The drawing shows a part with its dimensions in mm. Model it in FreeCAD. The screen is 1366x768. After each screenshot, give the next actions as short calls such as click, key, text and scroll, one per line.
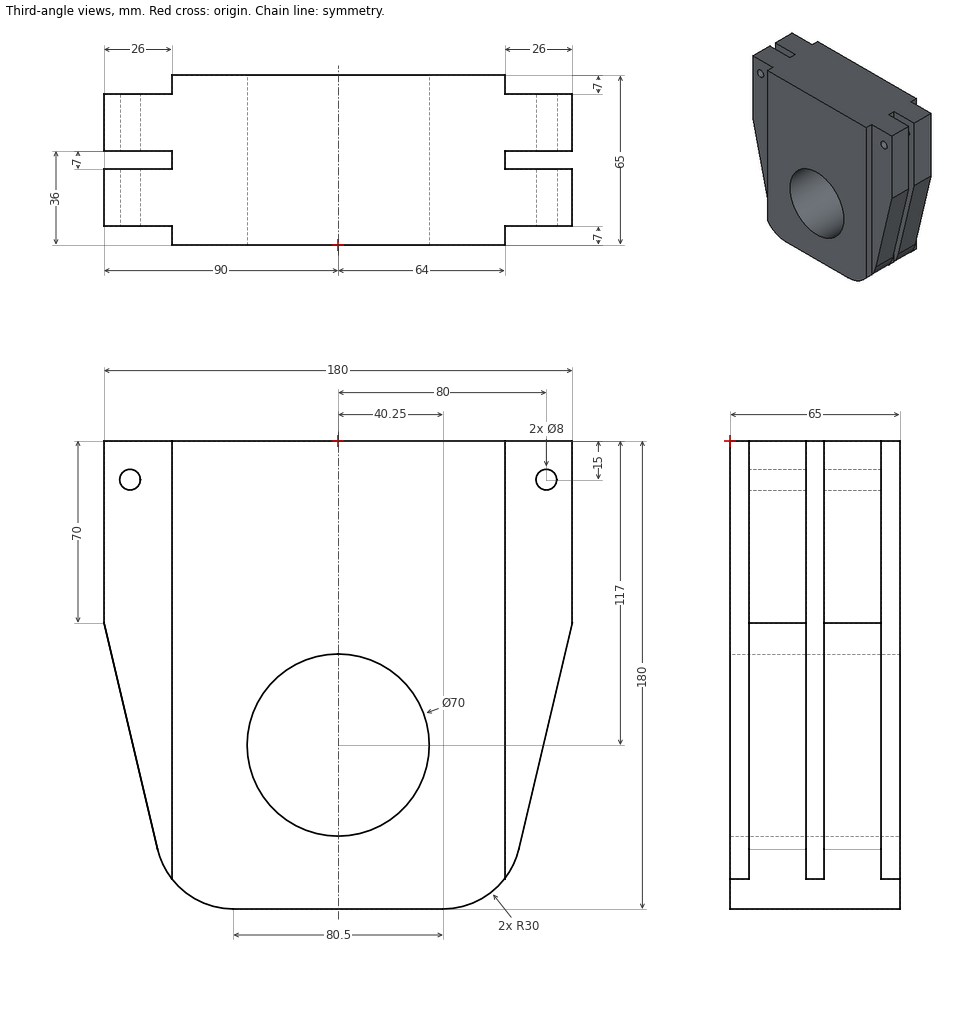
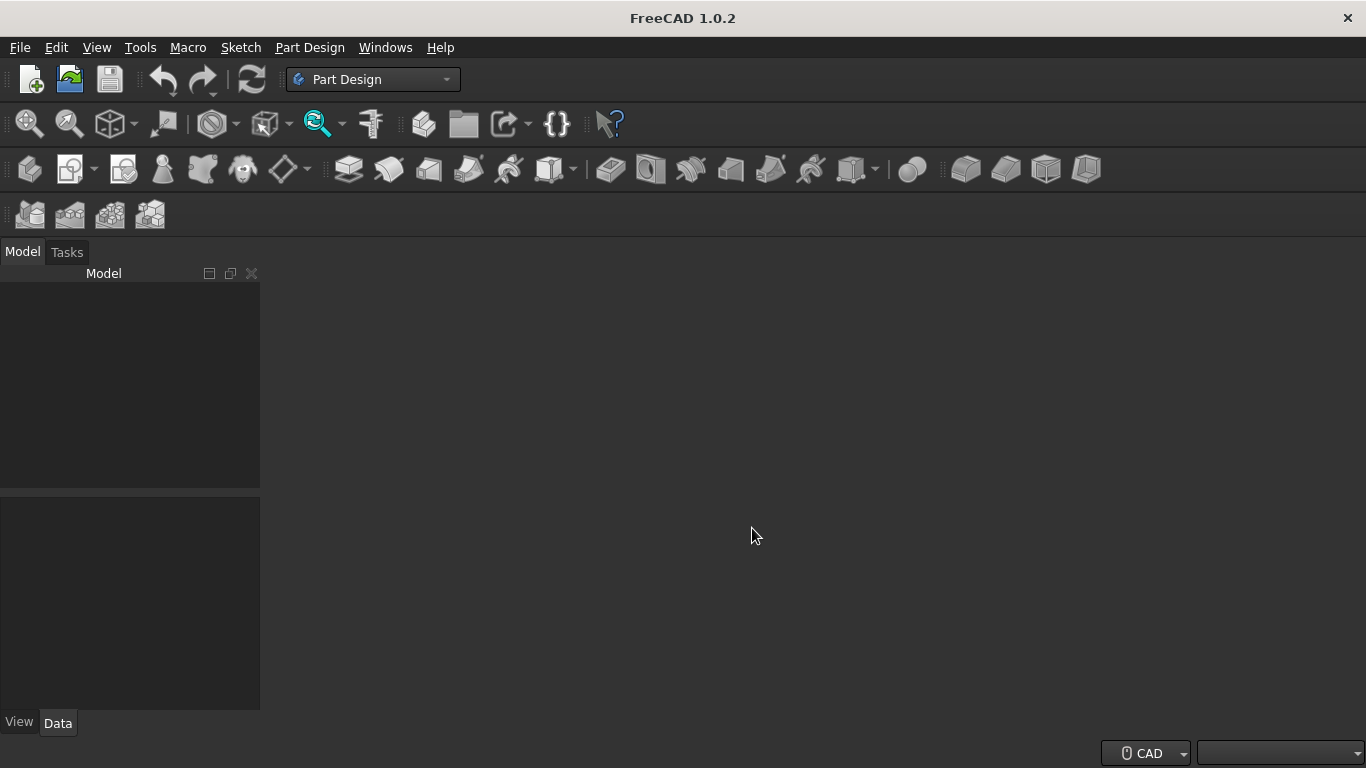
click(30, 80)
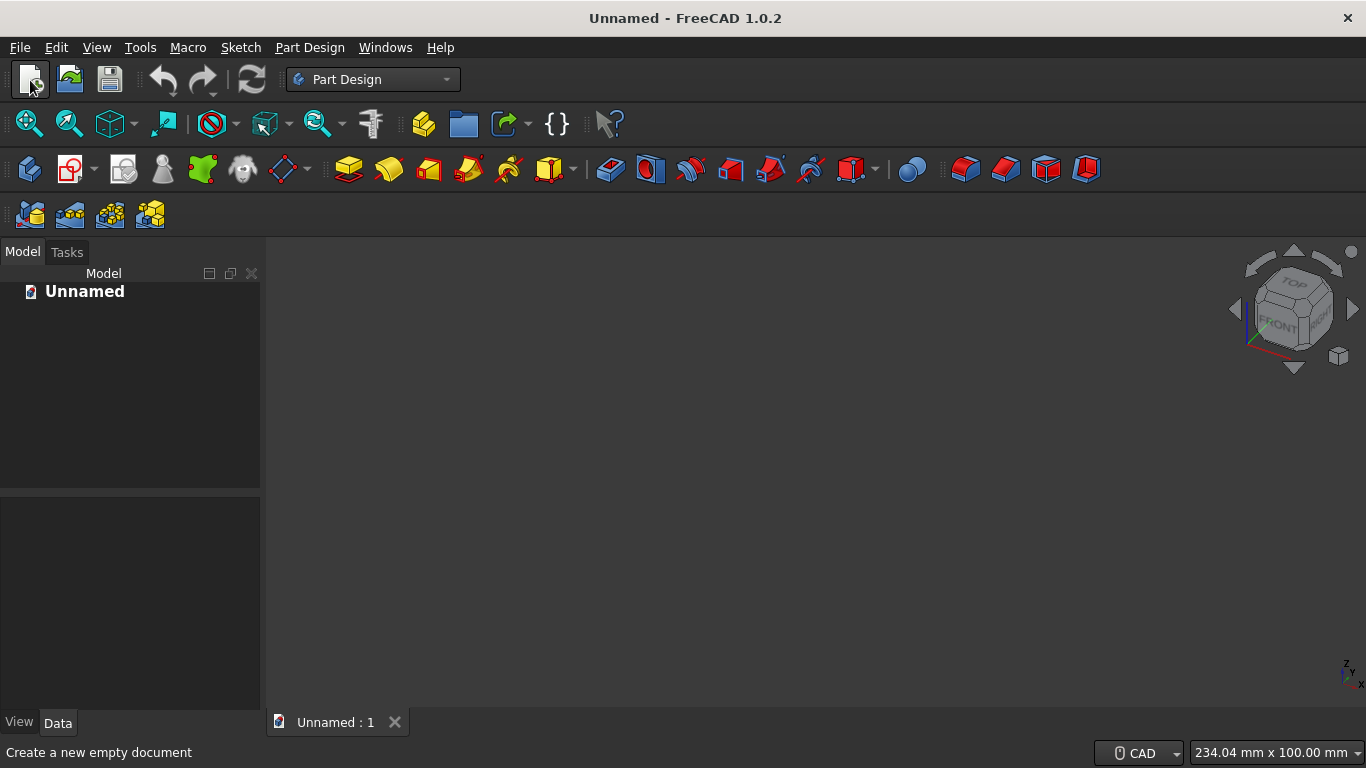
click(70, 170)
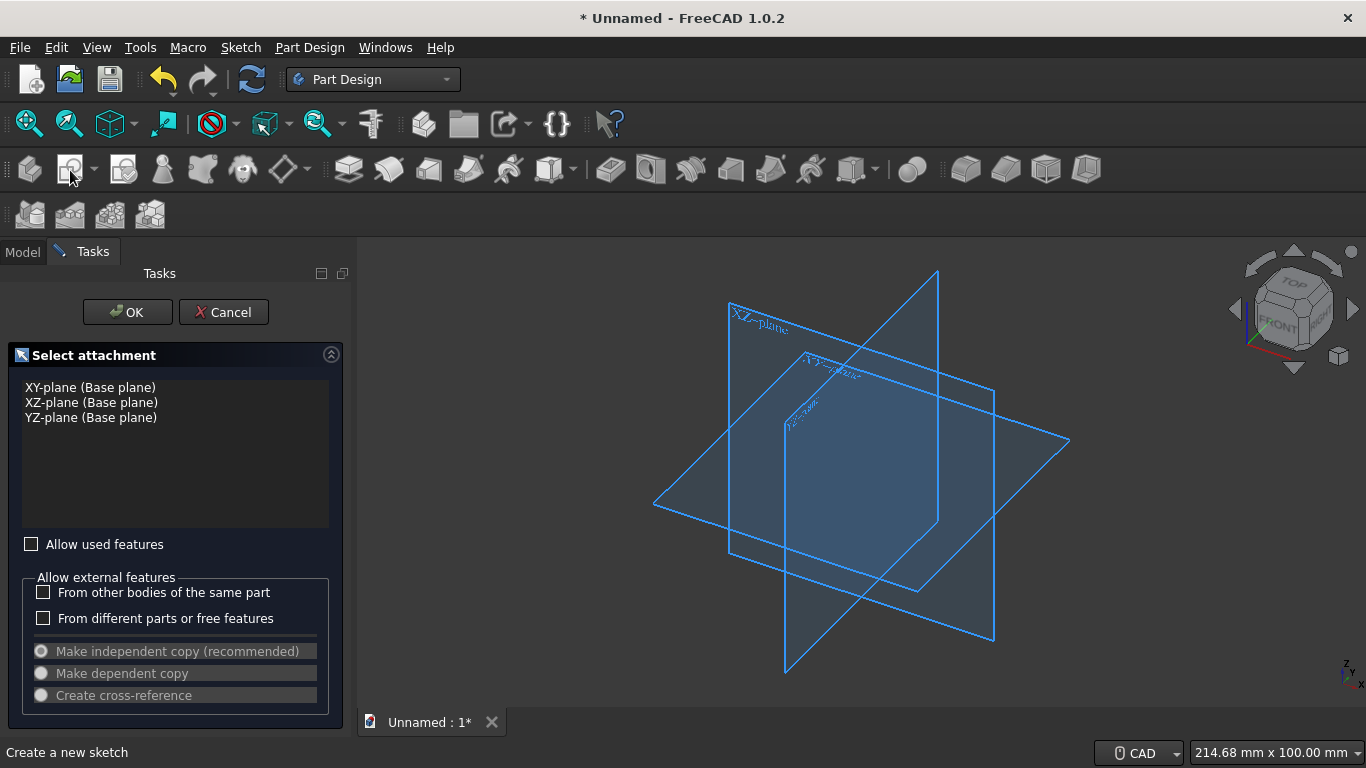
click(82, 402)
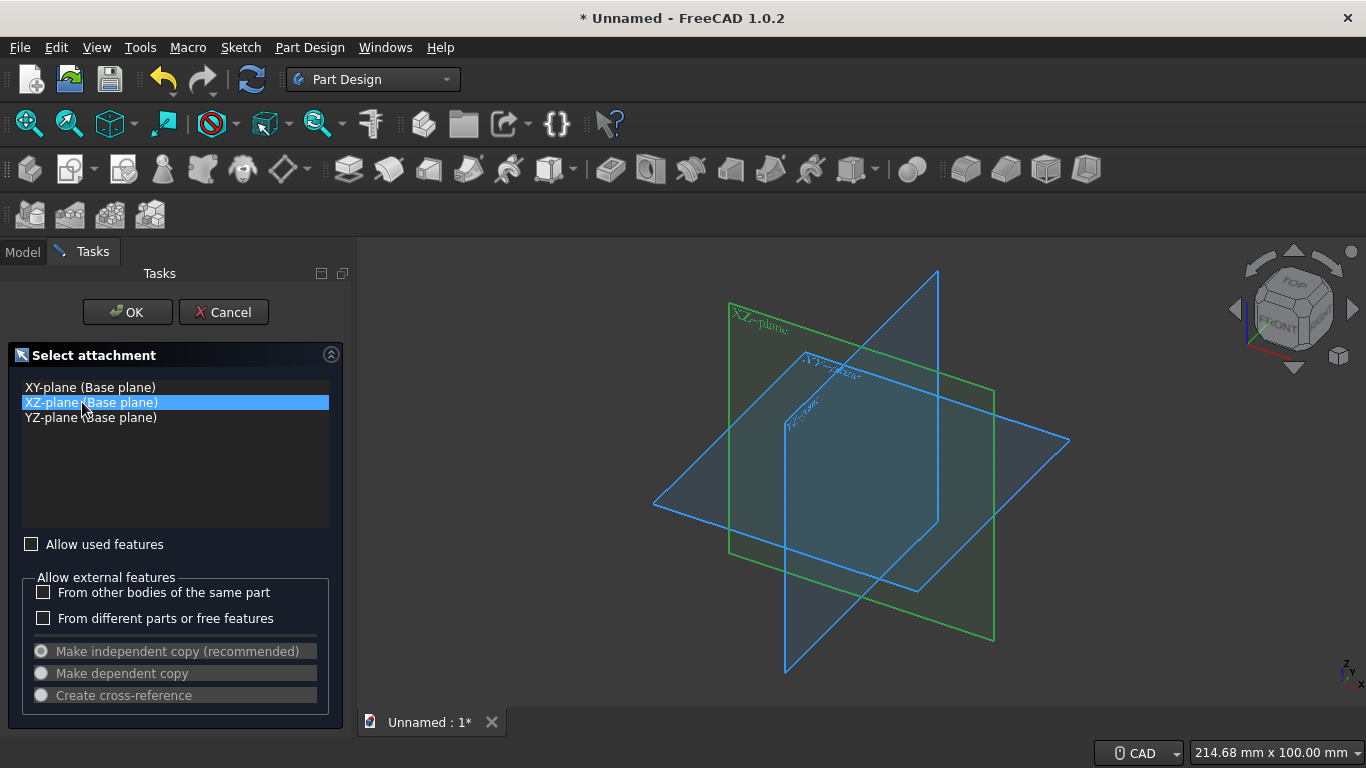
click(128, 312)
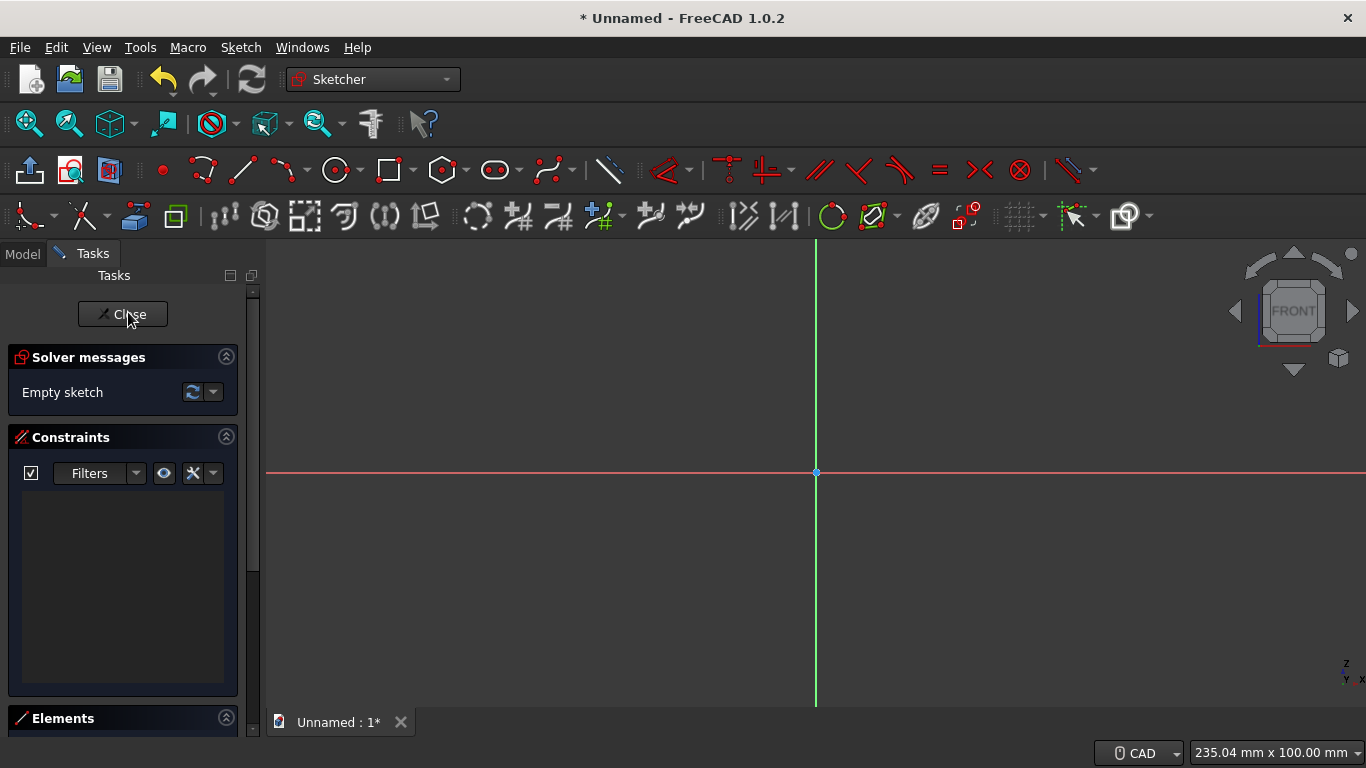
scroll(708, 267, down, 5)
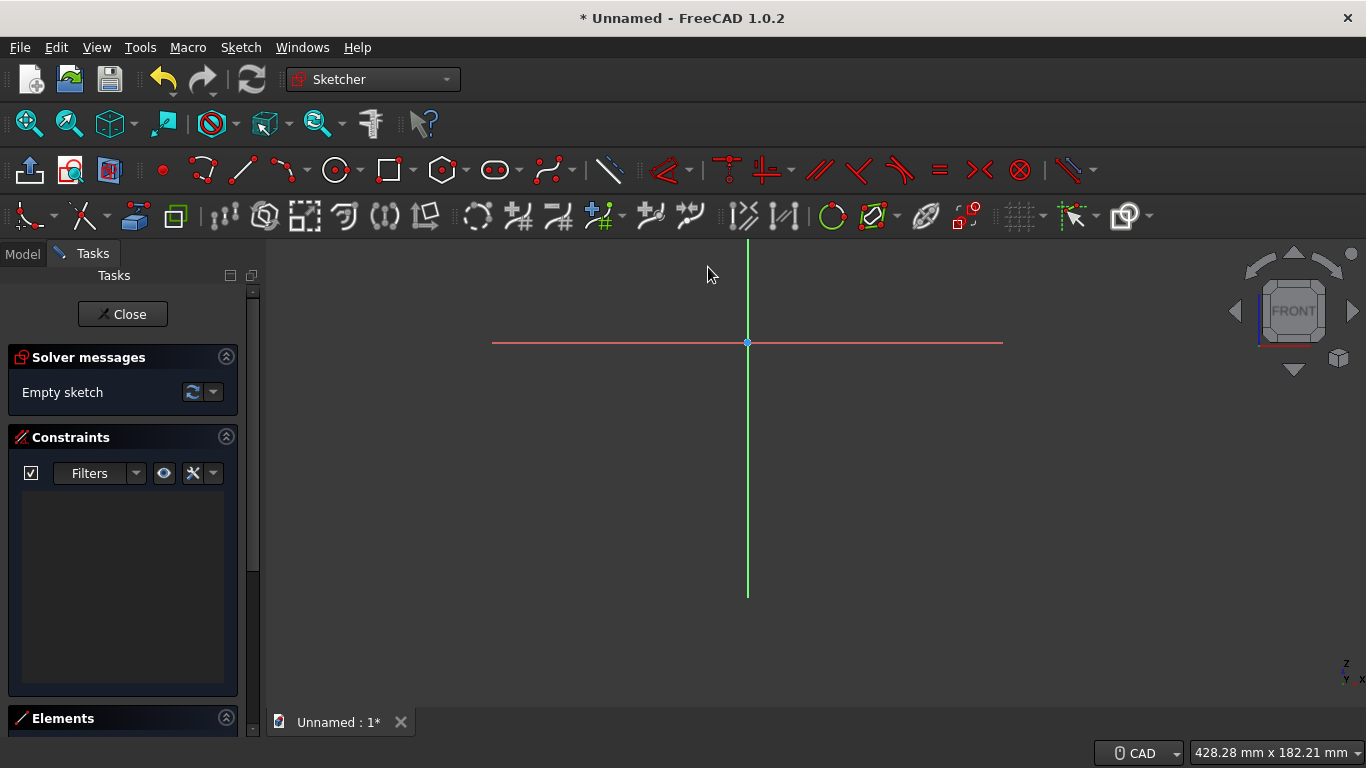
click(244, 170)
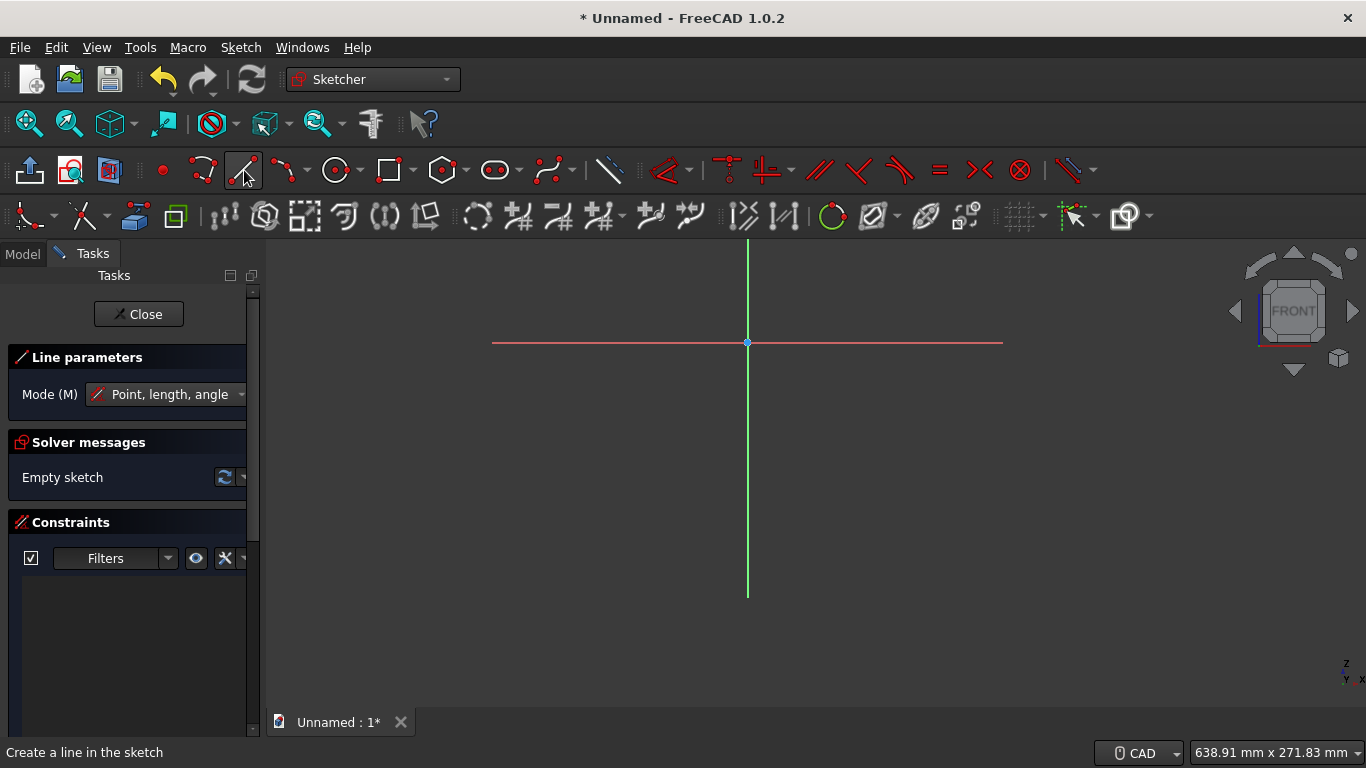
click(817, 653)
click(679, 653)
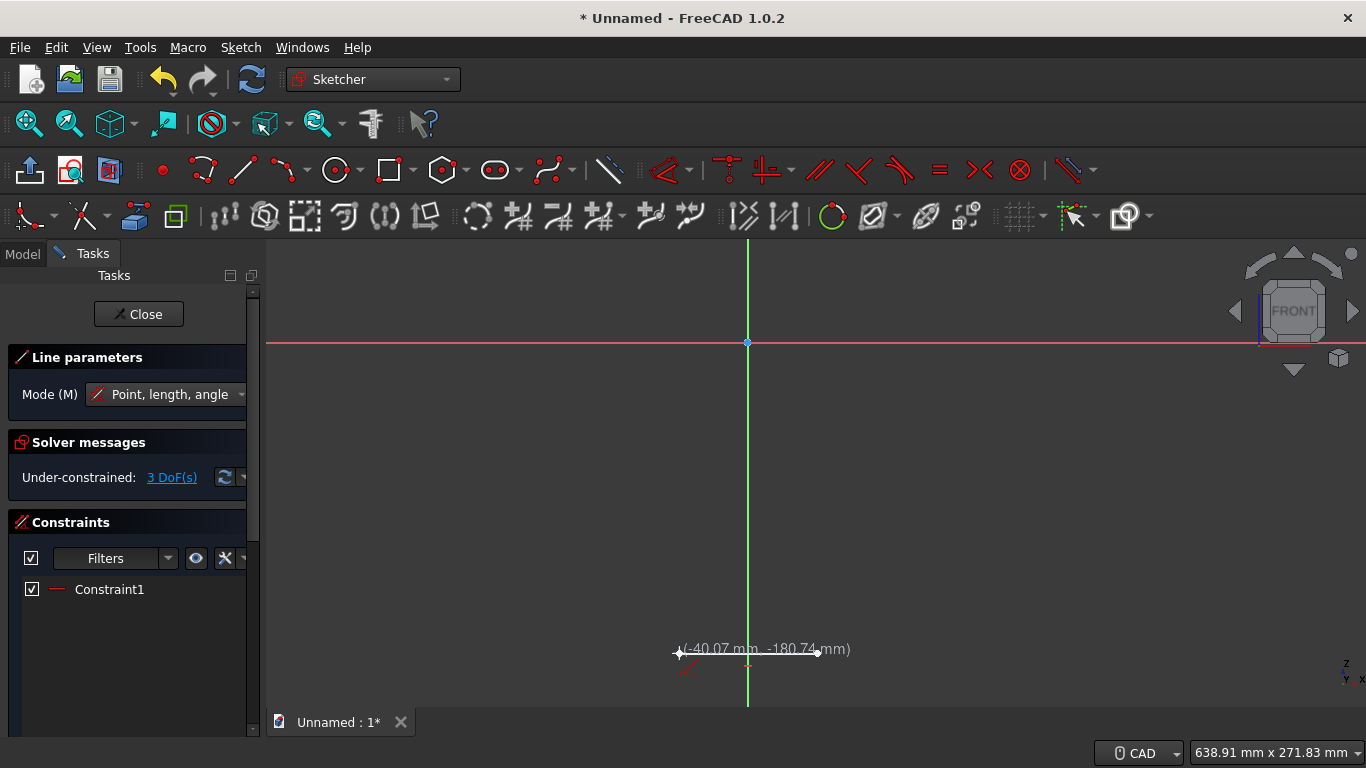
click(204, 170)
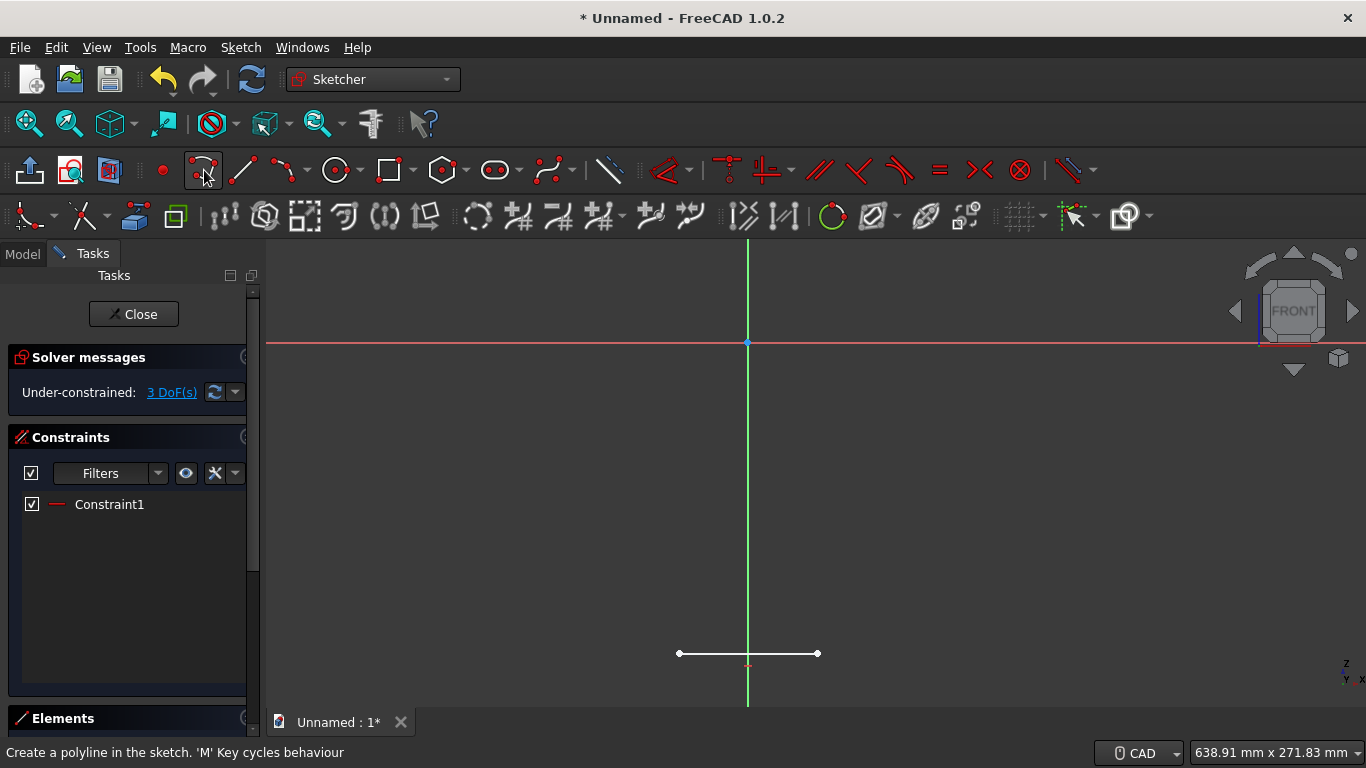
click(628, 613)
click(593, 463)
click(593, 343)
click(903, 352)
click(903, 463)
click(868, 613)
right_click(868, 613)